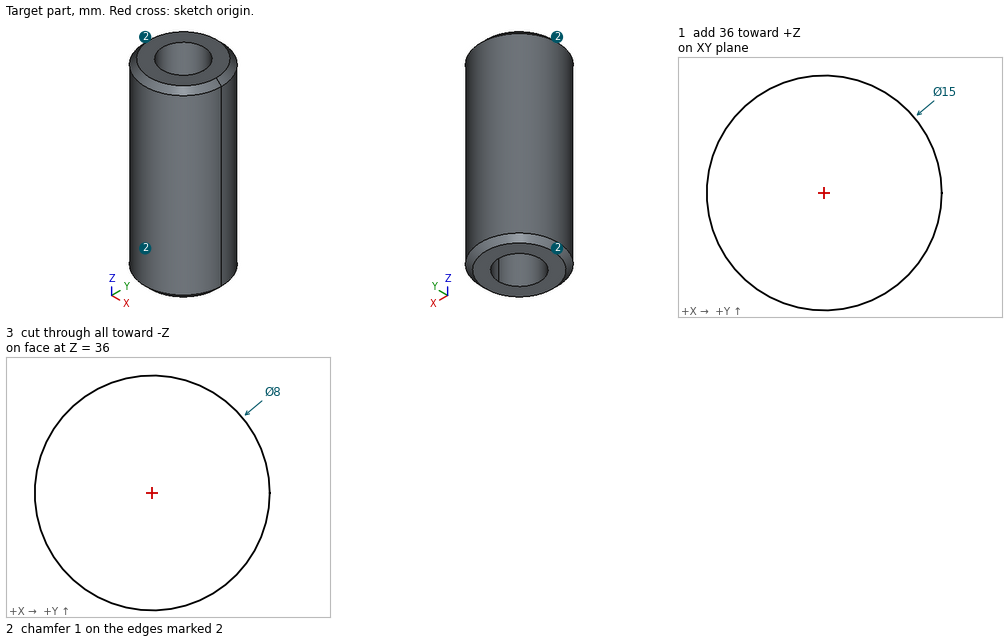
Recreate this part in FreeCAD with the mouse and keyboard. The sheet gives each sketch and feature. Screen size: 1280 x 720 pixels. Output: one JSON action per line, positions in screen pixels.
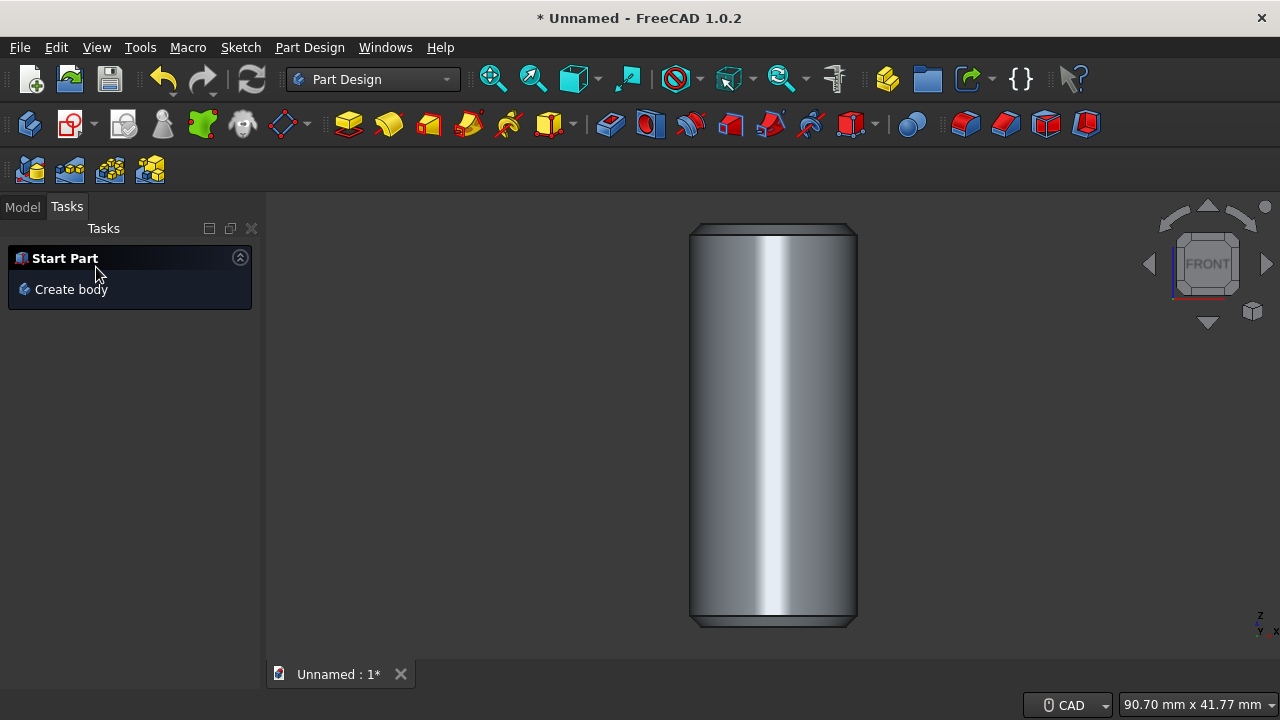
{"action": "key", "text": "0"}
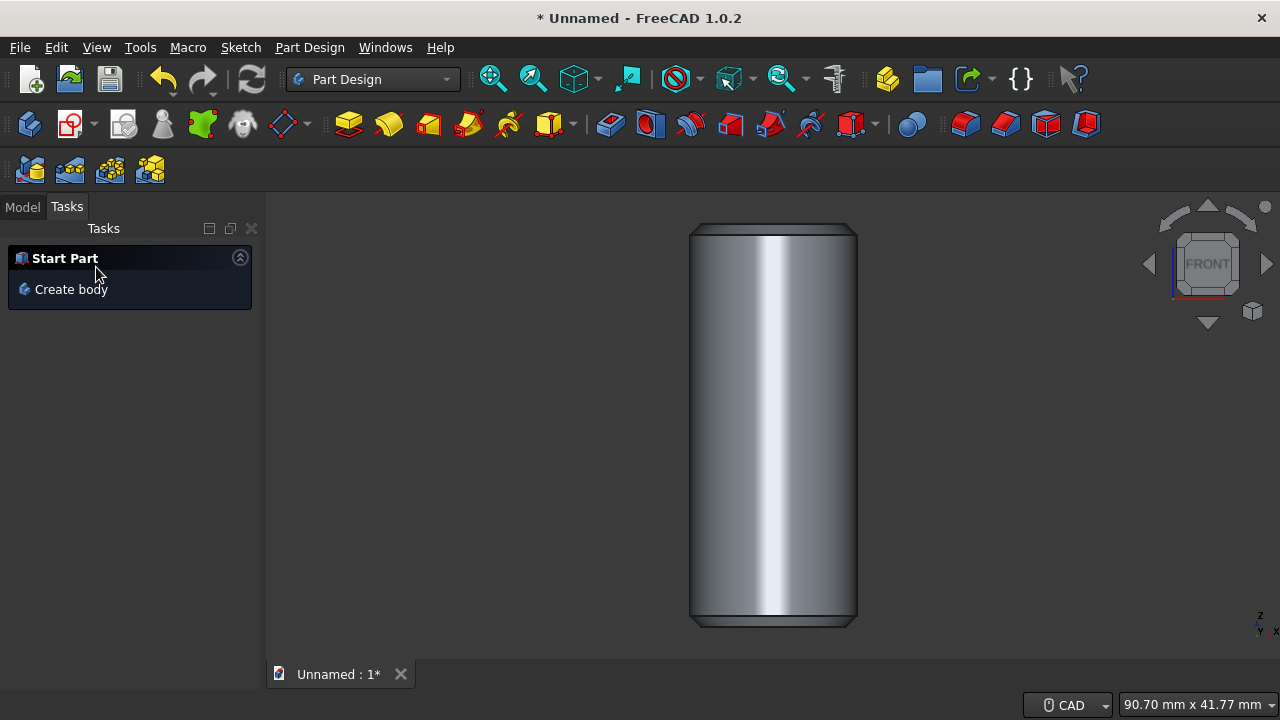
{"action": "left_click", "coordinate": [773, 260]}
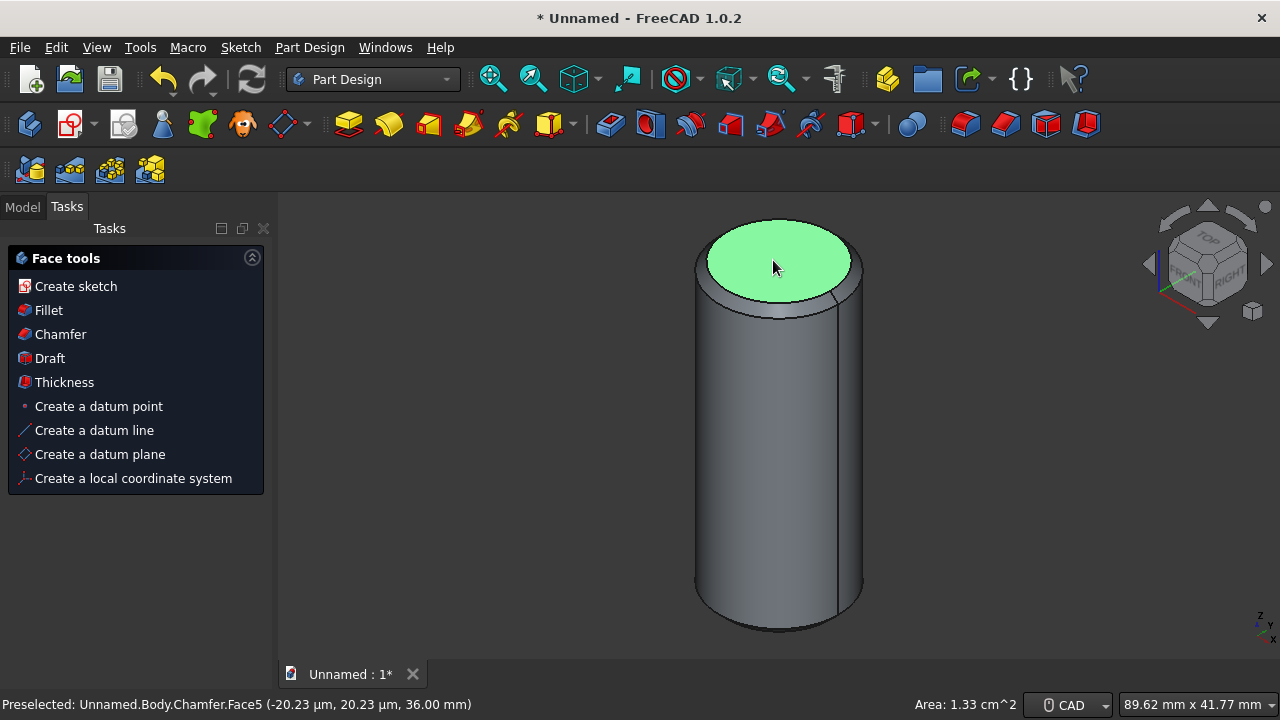
{"action": "left_click", "coordinate": [70, 124]}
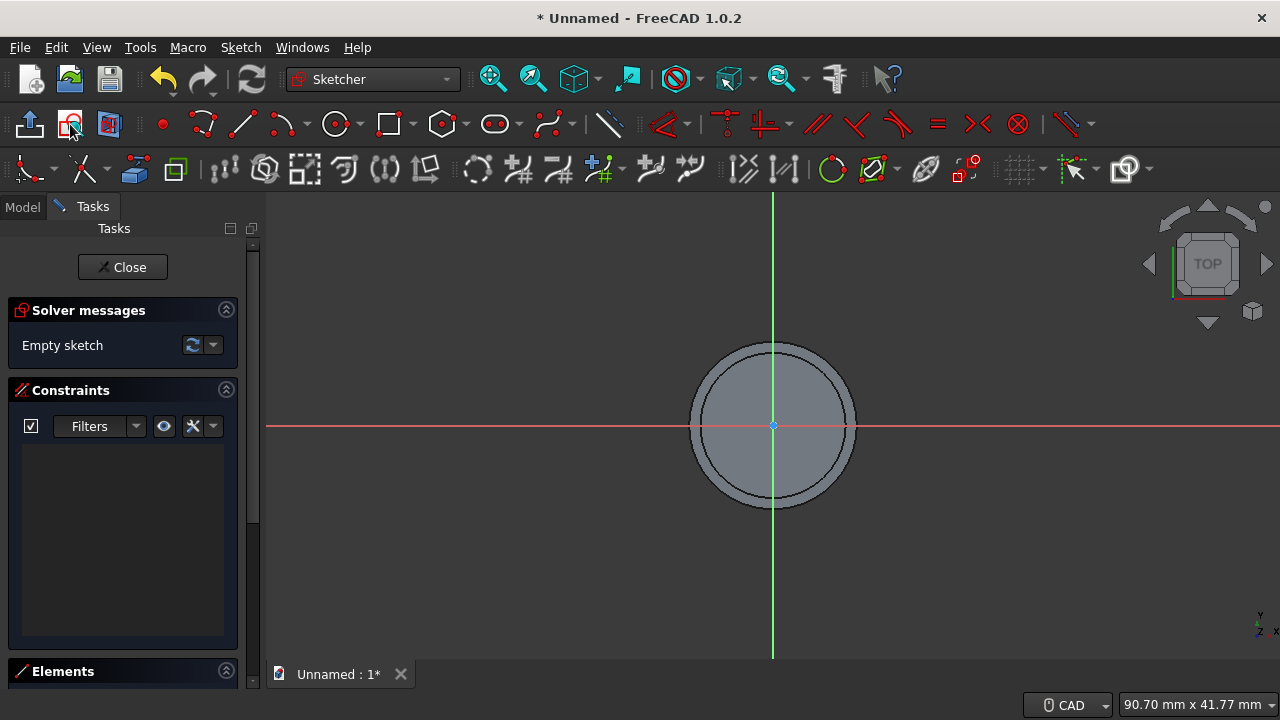
{"action": "scroll", "coordinate": [803, 426], "scroll_direction": "up", "scroll_amount": 6}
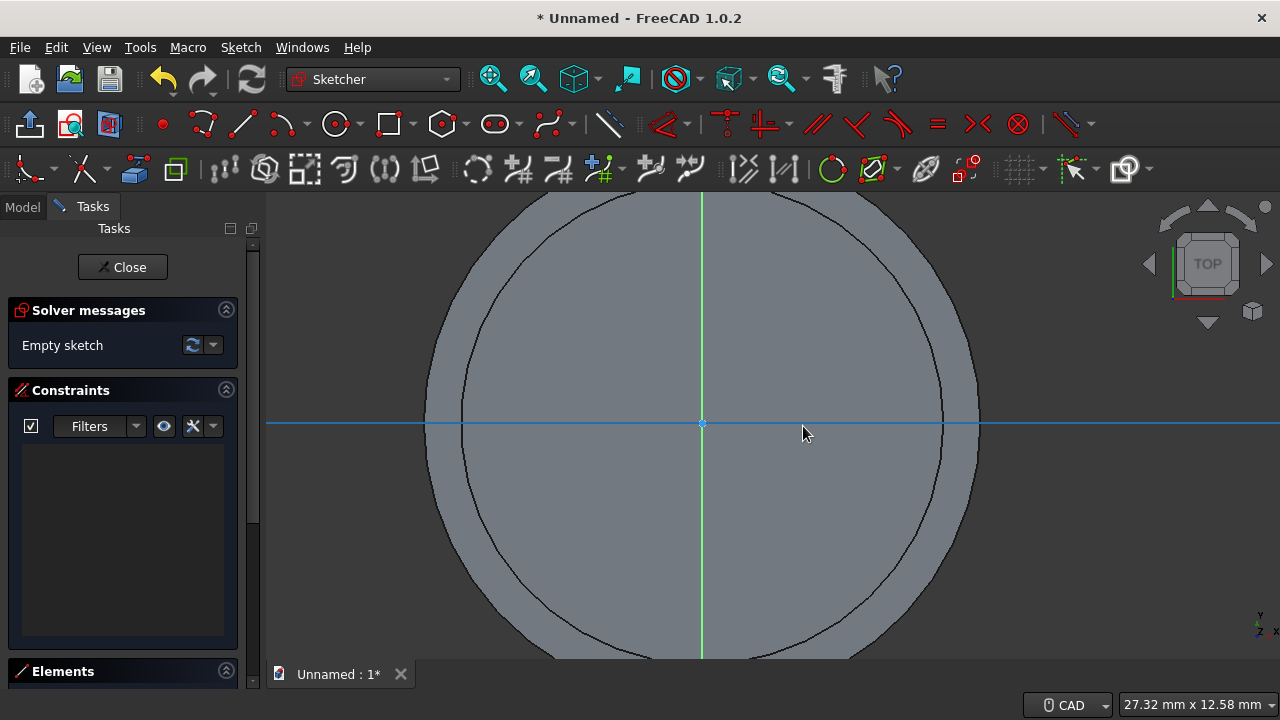
{"action": "left_click", "coordinate": [336, 124]}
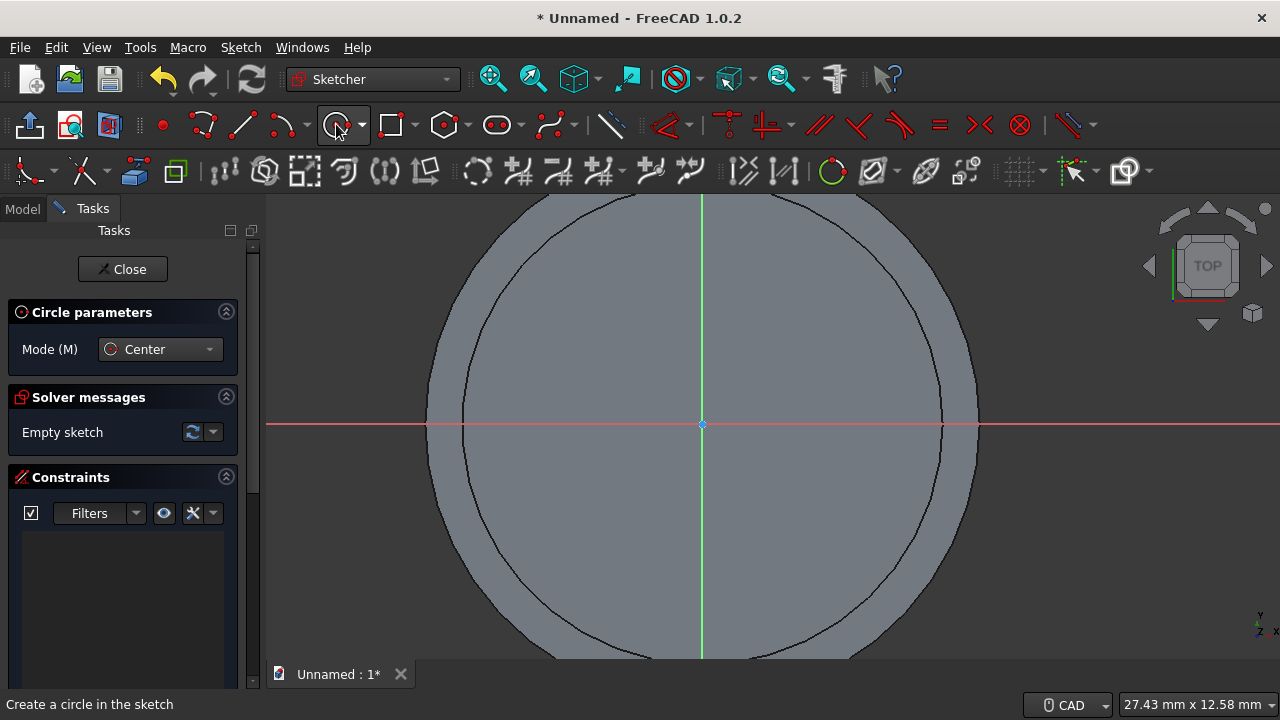
{"action": "left_click", "coordinate": [702, 424]}
{"action": "mouse_move", "coordinate": [807, 320]}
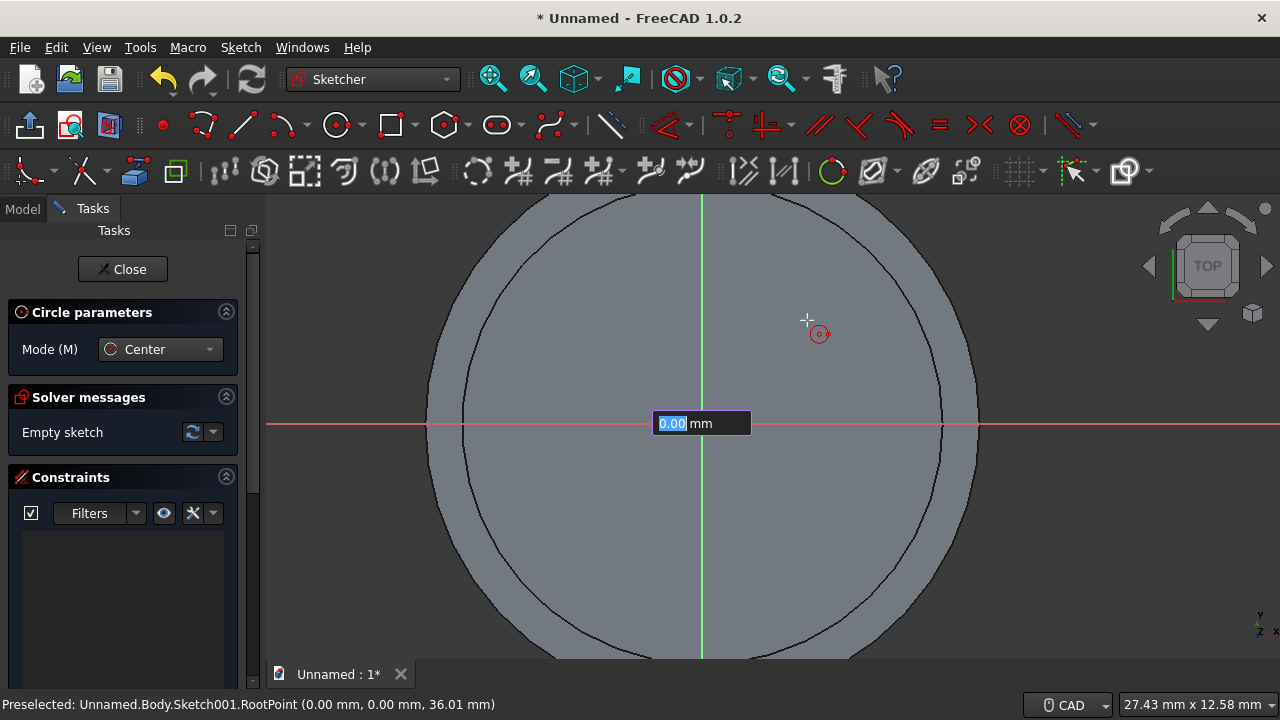
{"action": "type", "text": "8"}
{"action": "key", "text": "Return"}
{"action": "key", "text": "Escape"}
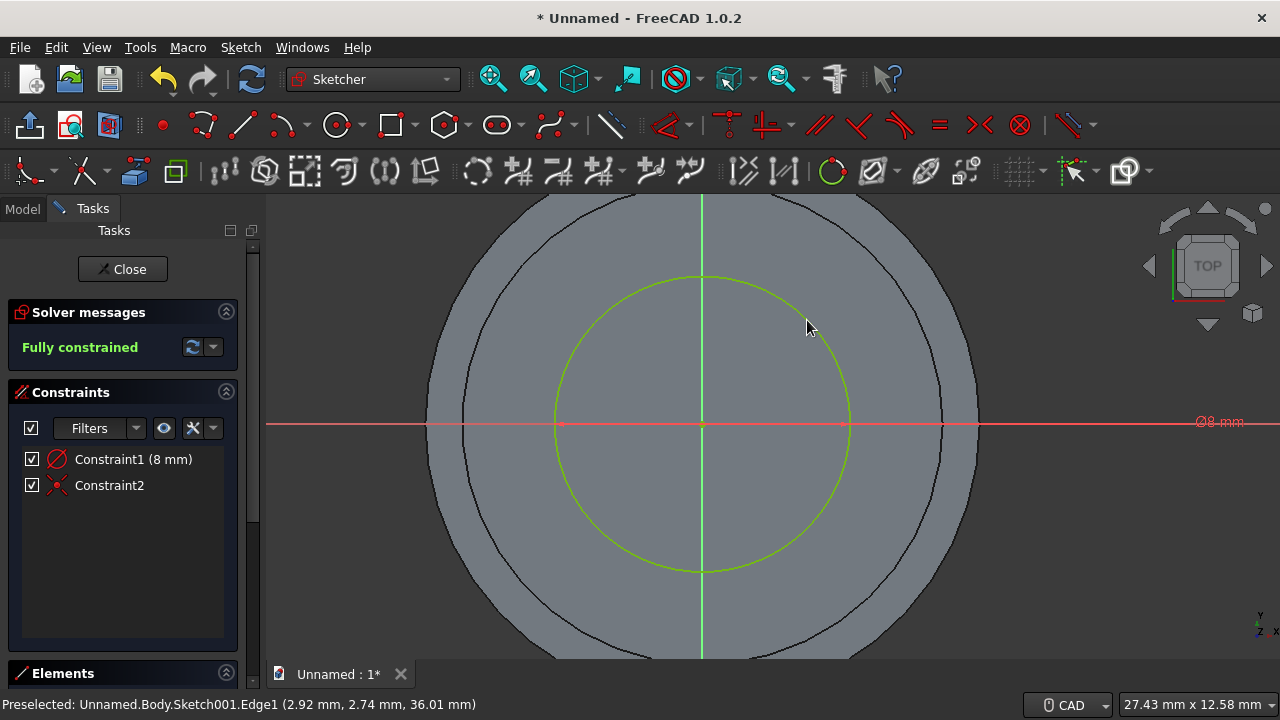
{"action": "left_click", "coordinate": [123, 269]}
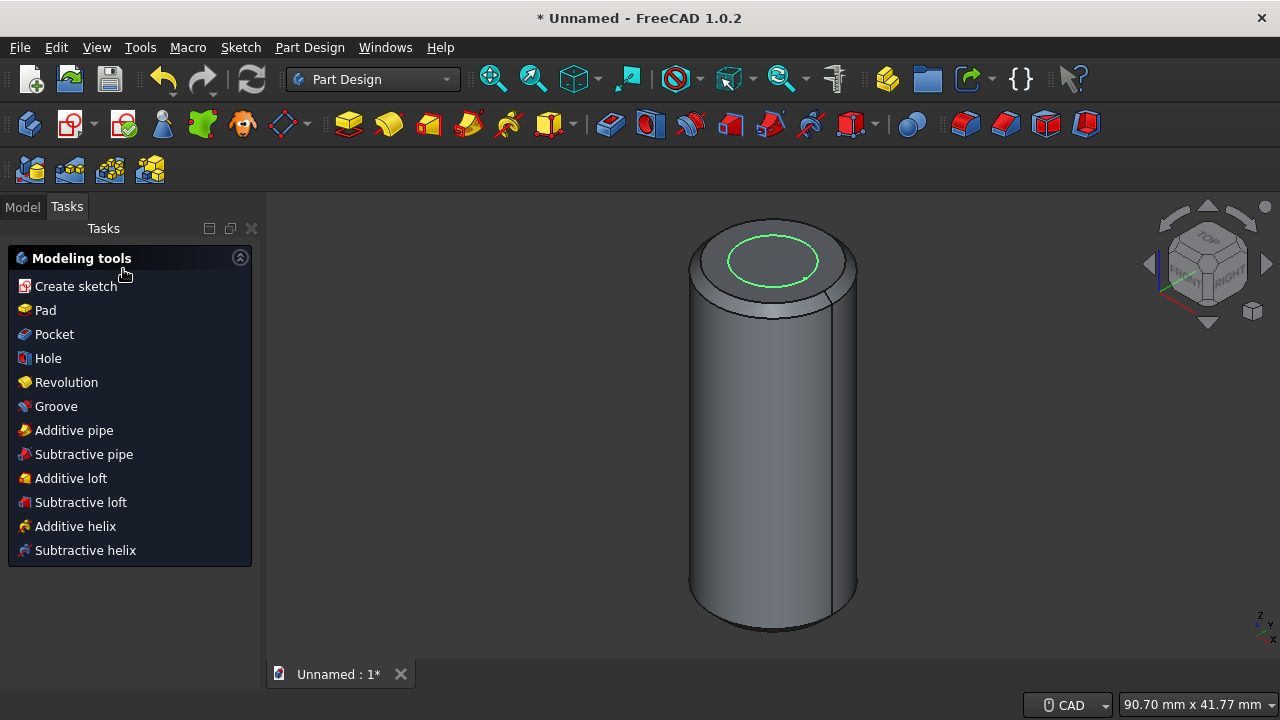
{"action": "left_click", "coordinate": [612, 124]}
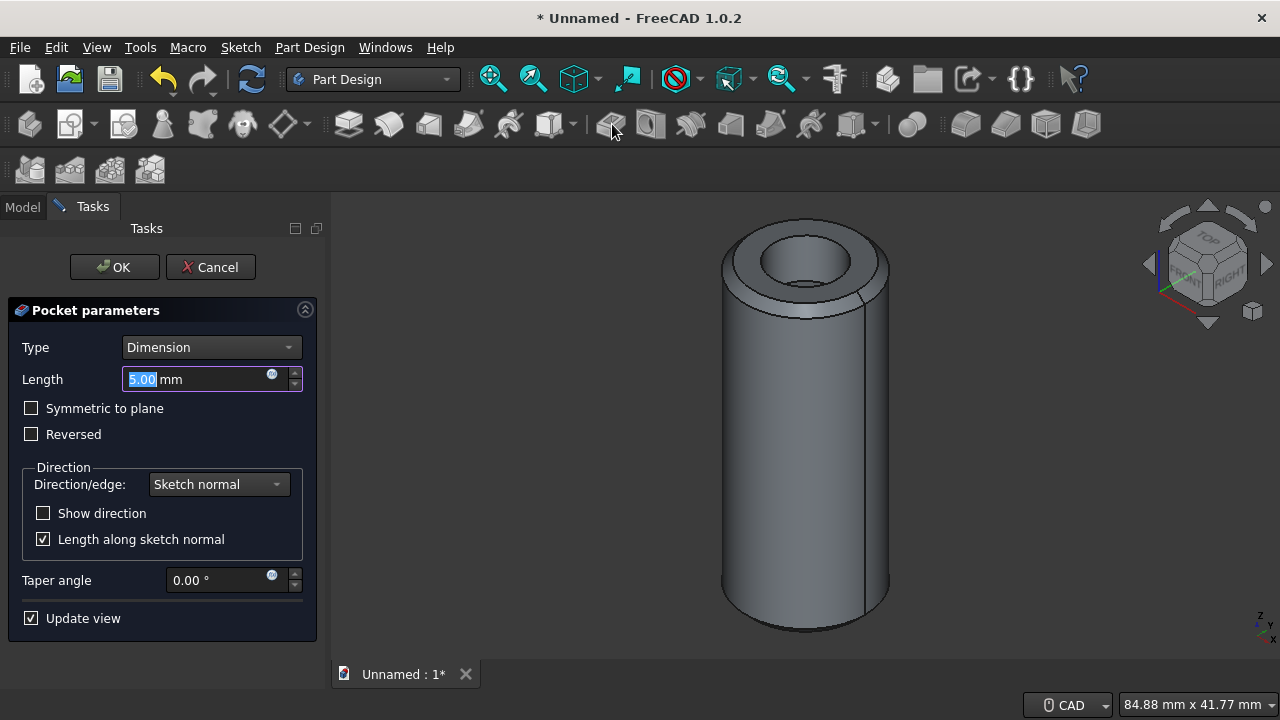
{"action": "left_click", "coordinate": [212, 348]}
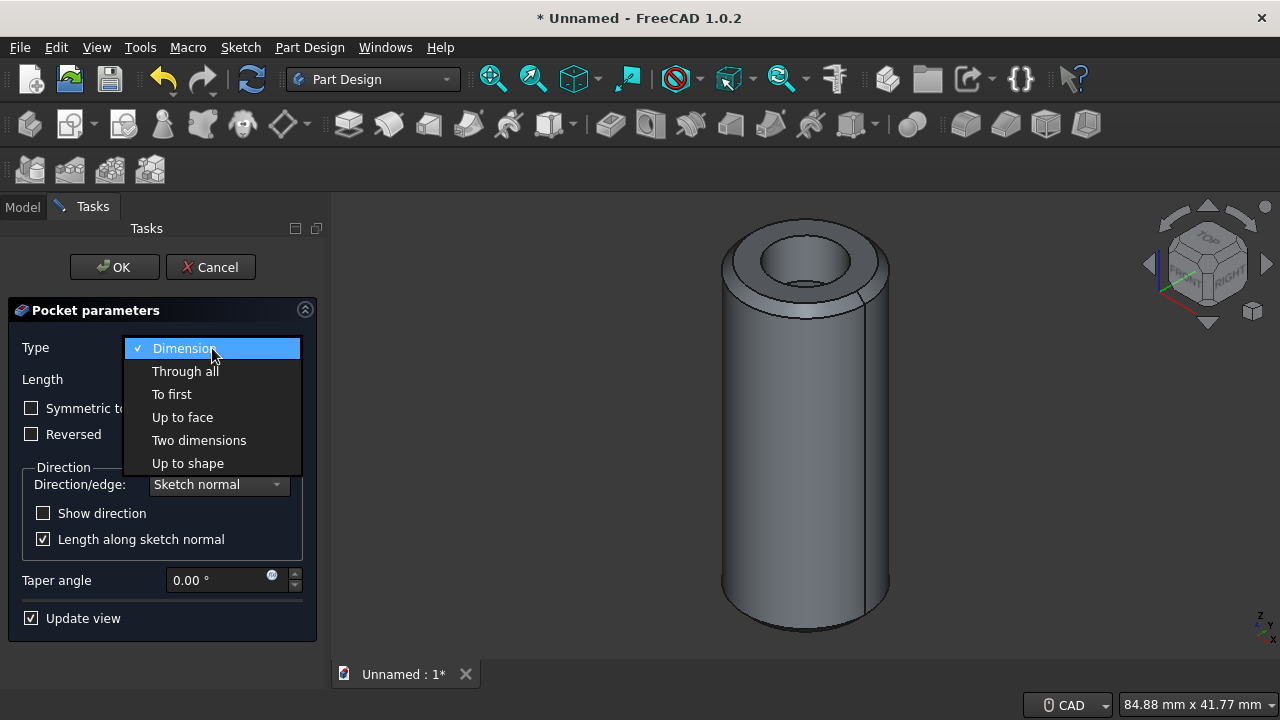
{"action": "left_click", "coordinate": [212, 372]}